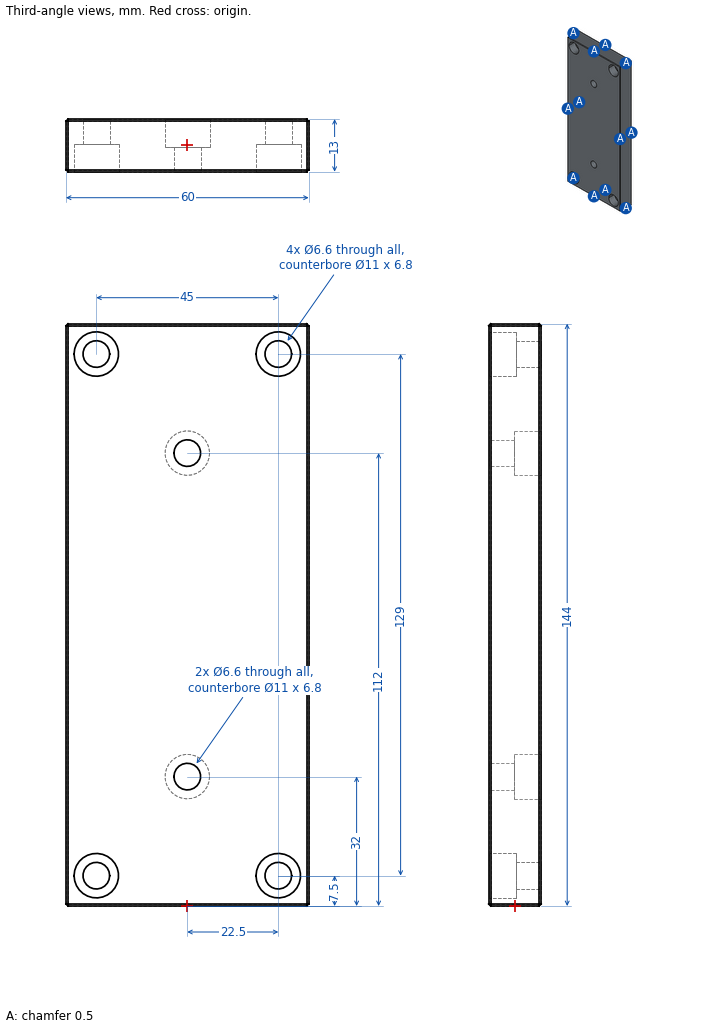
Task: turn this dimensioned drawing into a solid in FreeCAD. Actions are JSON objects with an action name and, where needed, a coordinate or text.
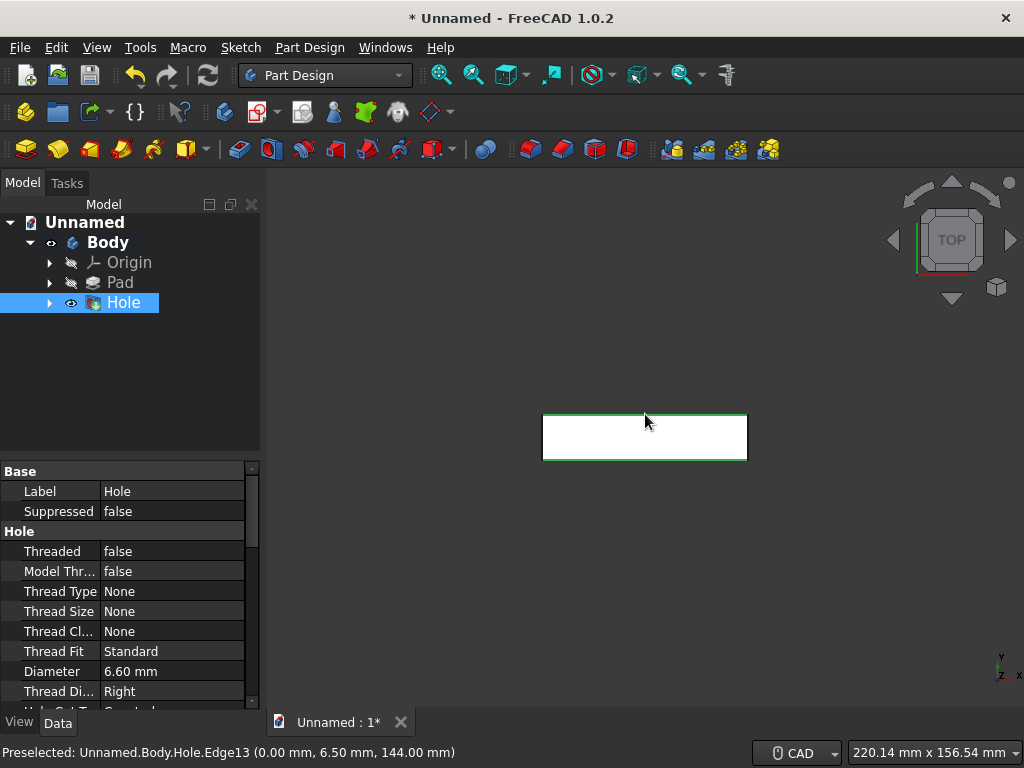
{"action": "key", "text": "1"}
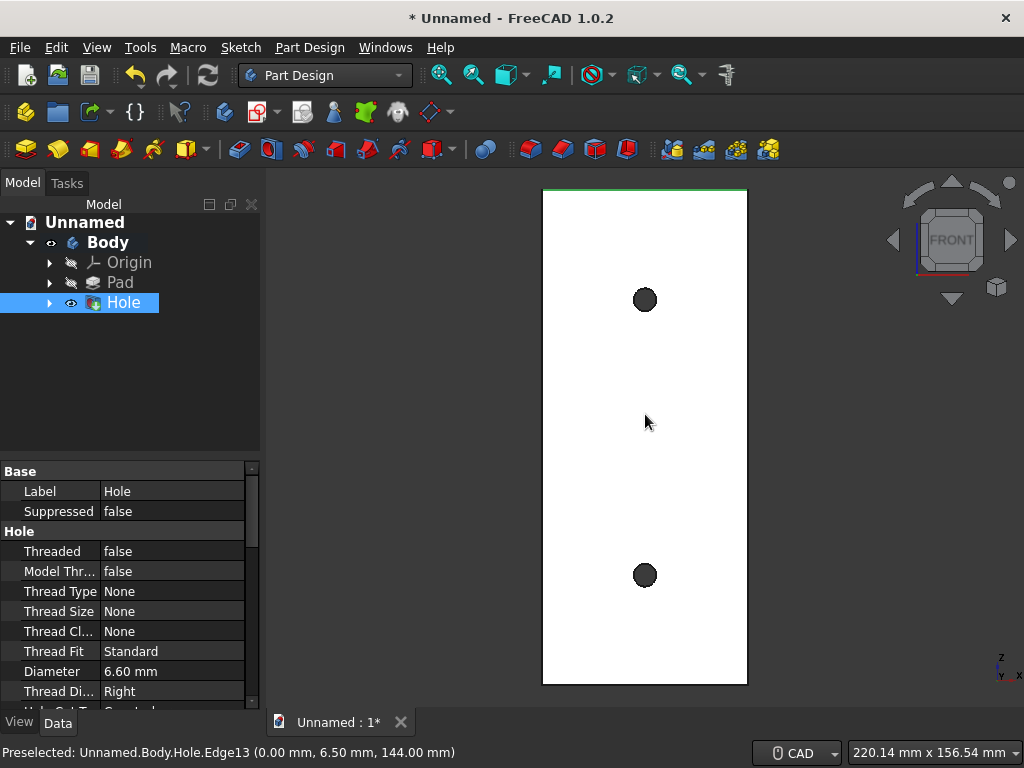
{"action": "key", "text": "3"}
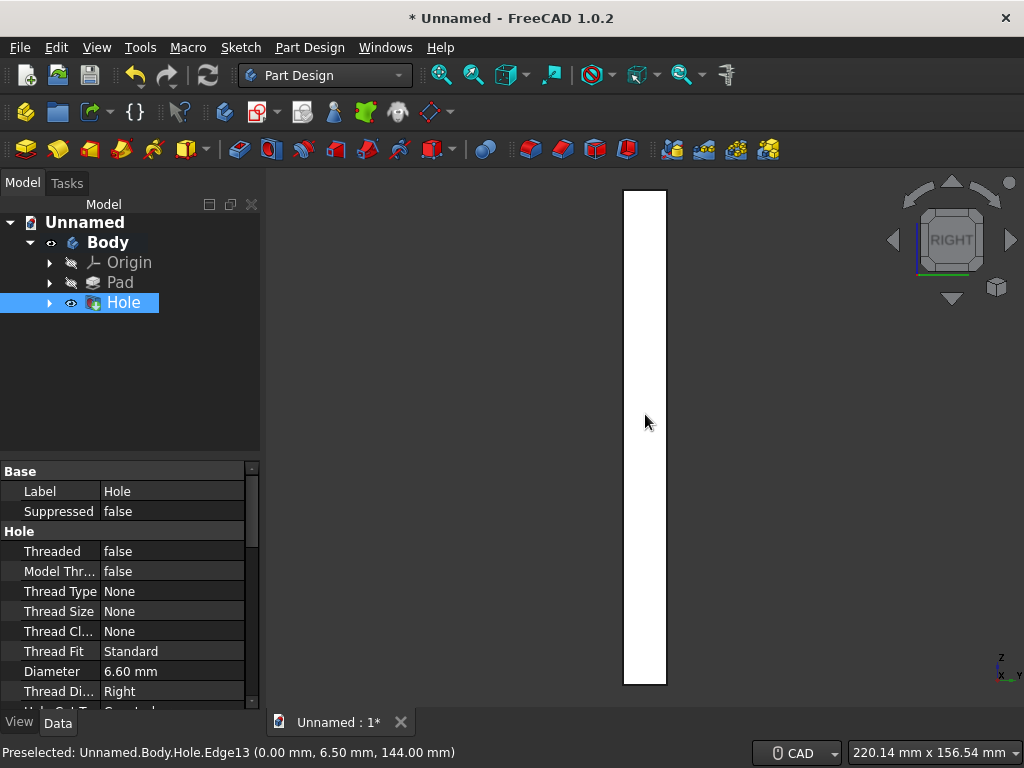
{"action": "key", "text": "5"}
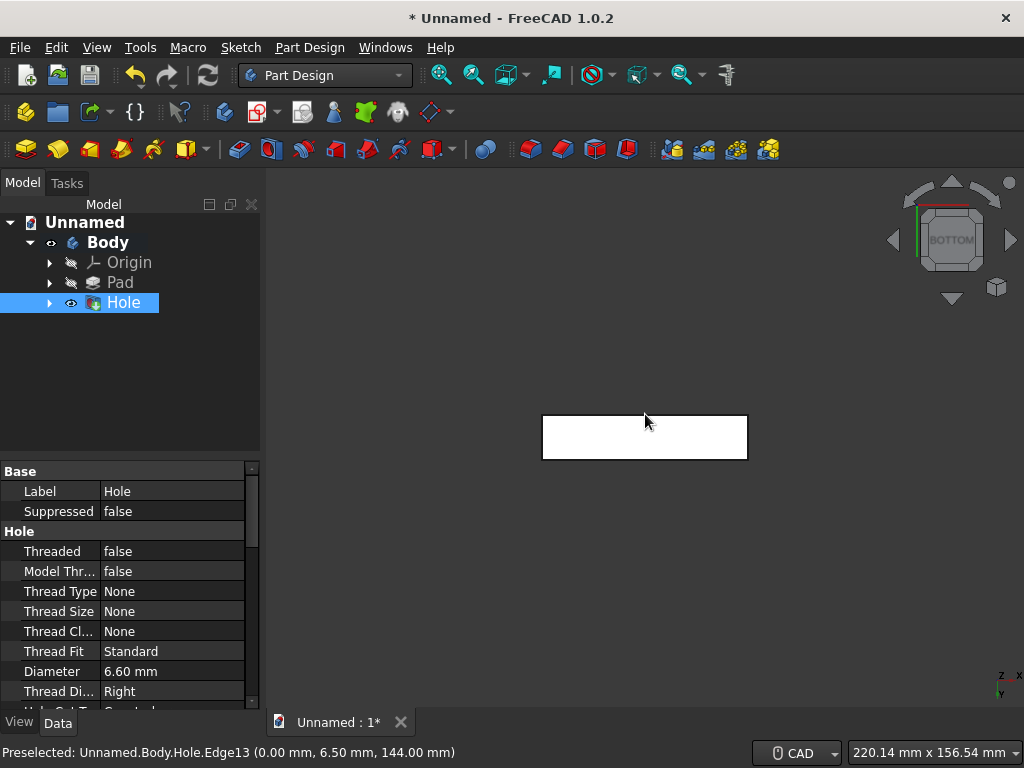
{"action": "key", "text": "v f"}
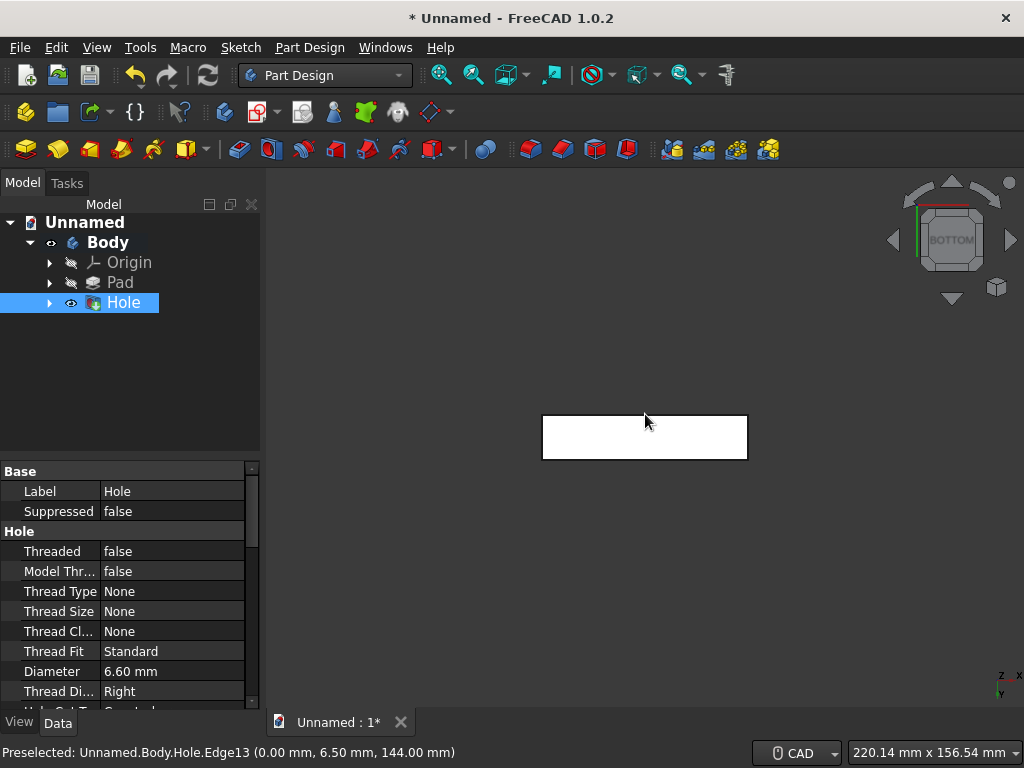
{"action": "left_click", "coordinate": [645, 414], "text": "ctrl"}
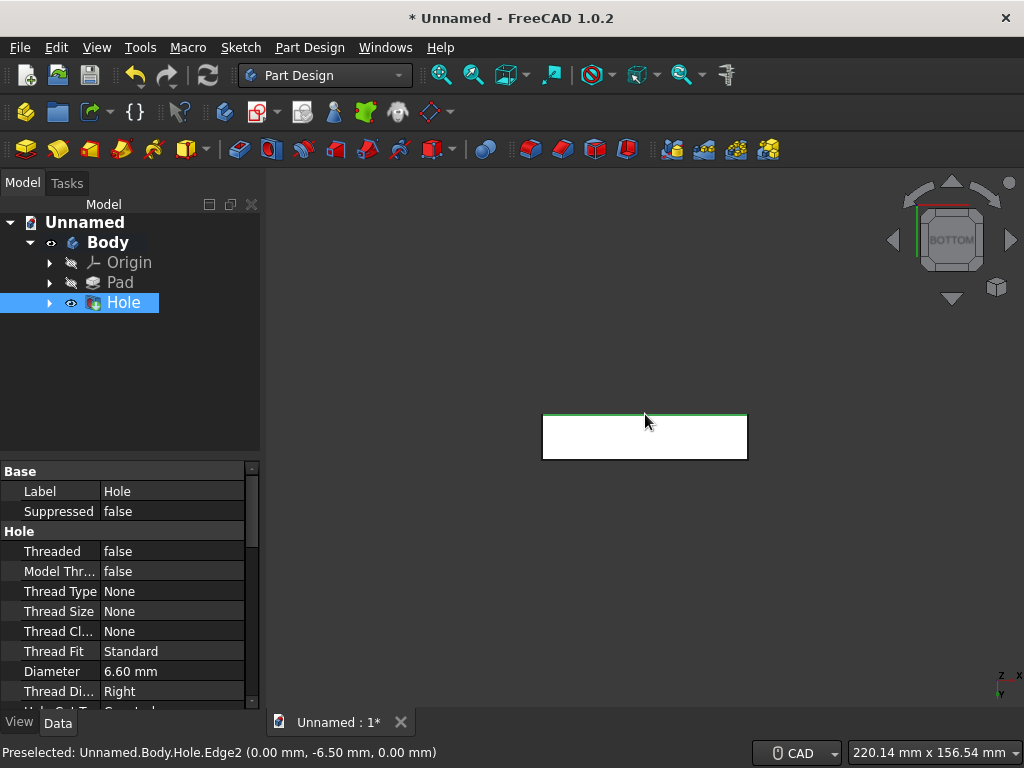
{"action": "left_click", "coordinate": [645, 459], "text": "ctrl"}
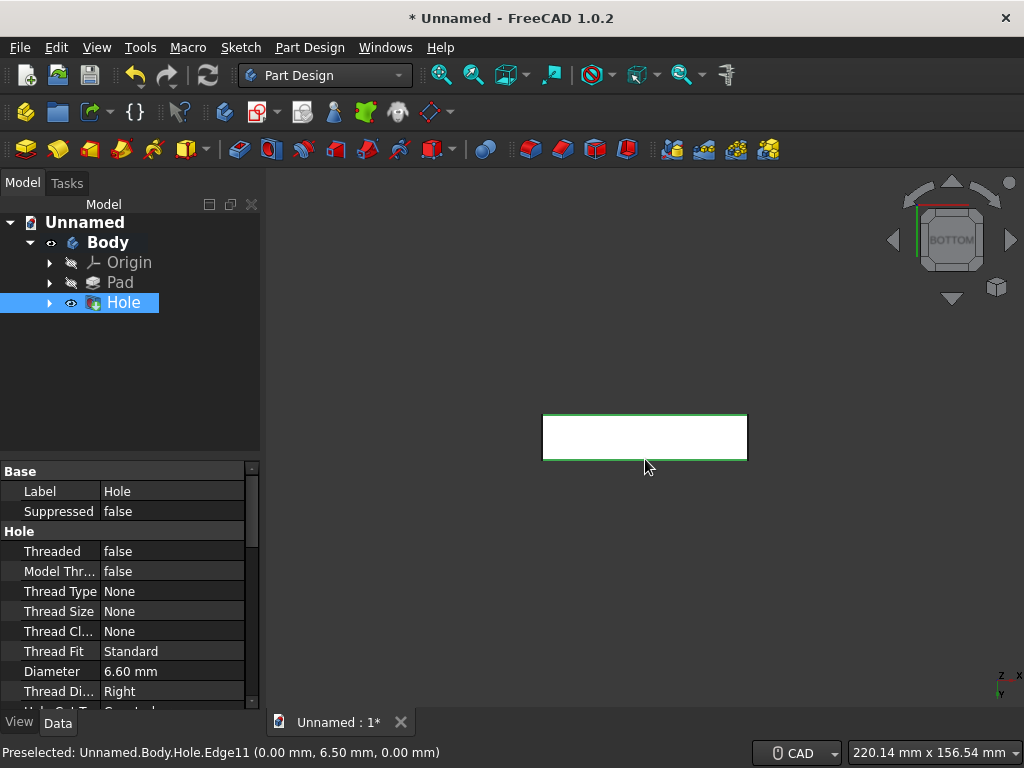
{"action": "key", "text": "4"}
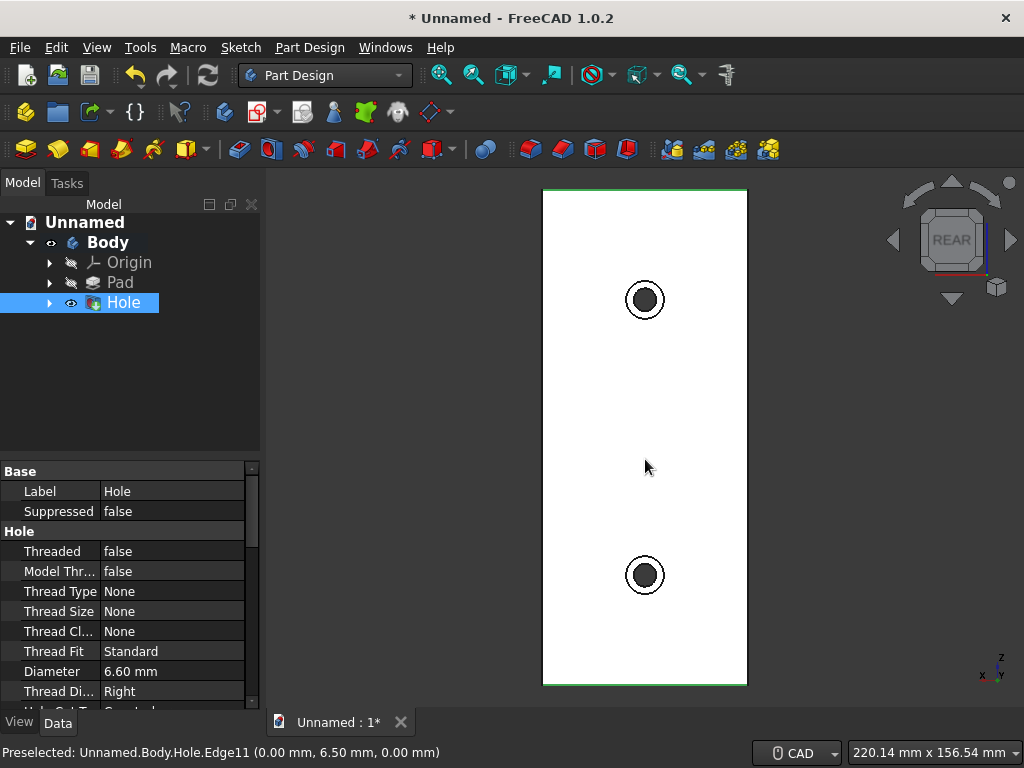
{"action": "key", "text": "6"}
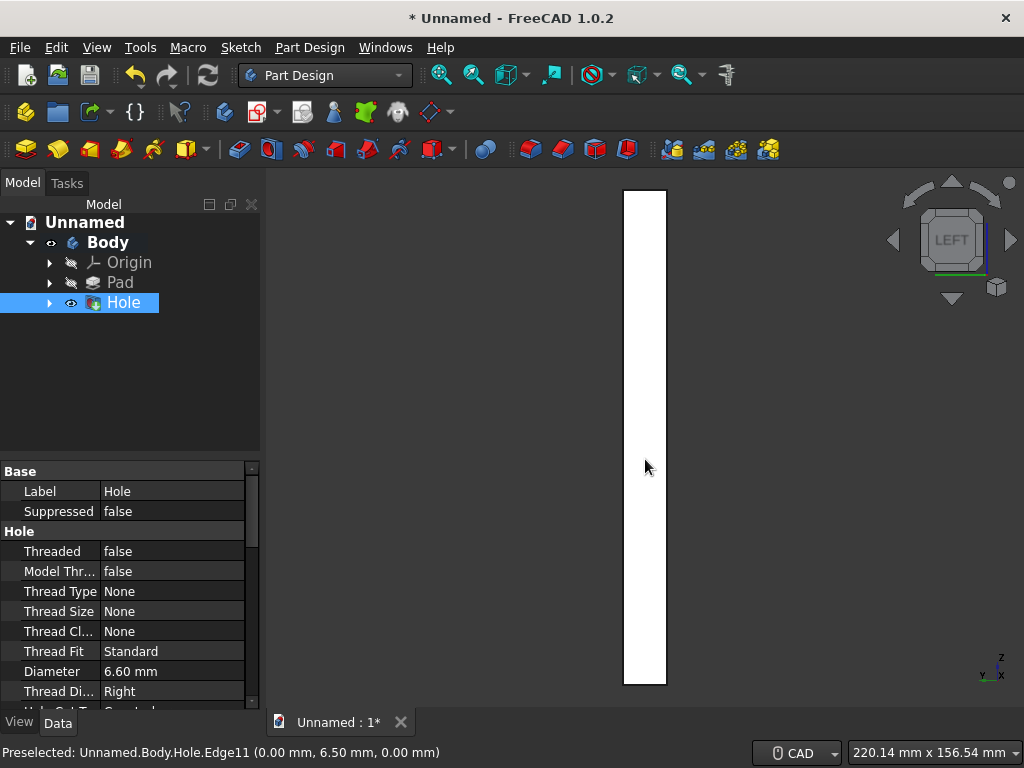
{"action": "left_click", "coordinate": [645, 224], "text": "ctrl"}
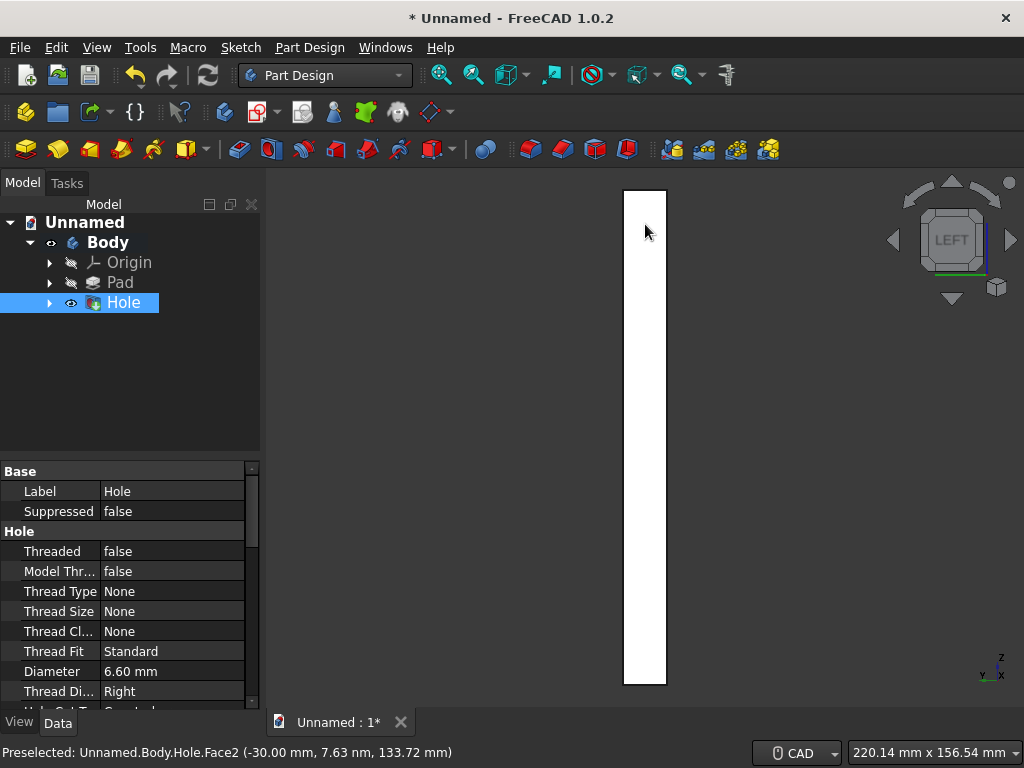
{"action": "left_click", "coordinate": [564, 150]}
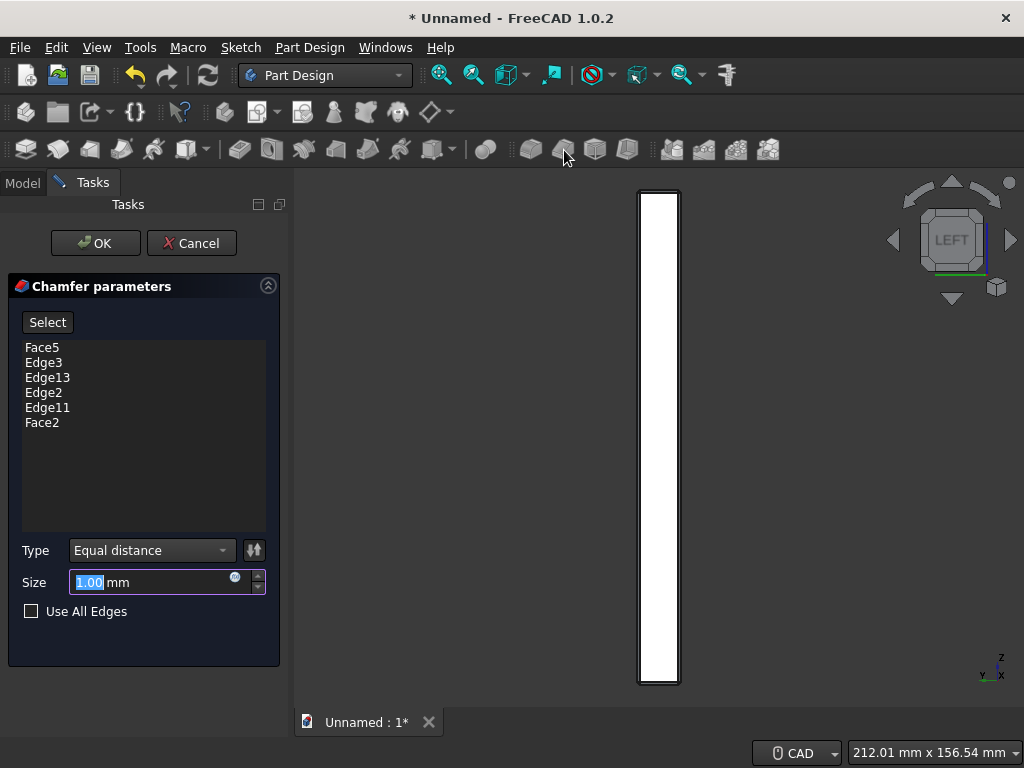
{"action": "type", "text": "0.5"}
{"action": "key", "text": "Tab"}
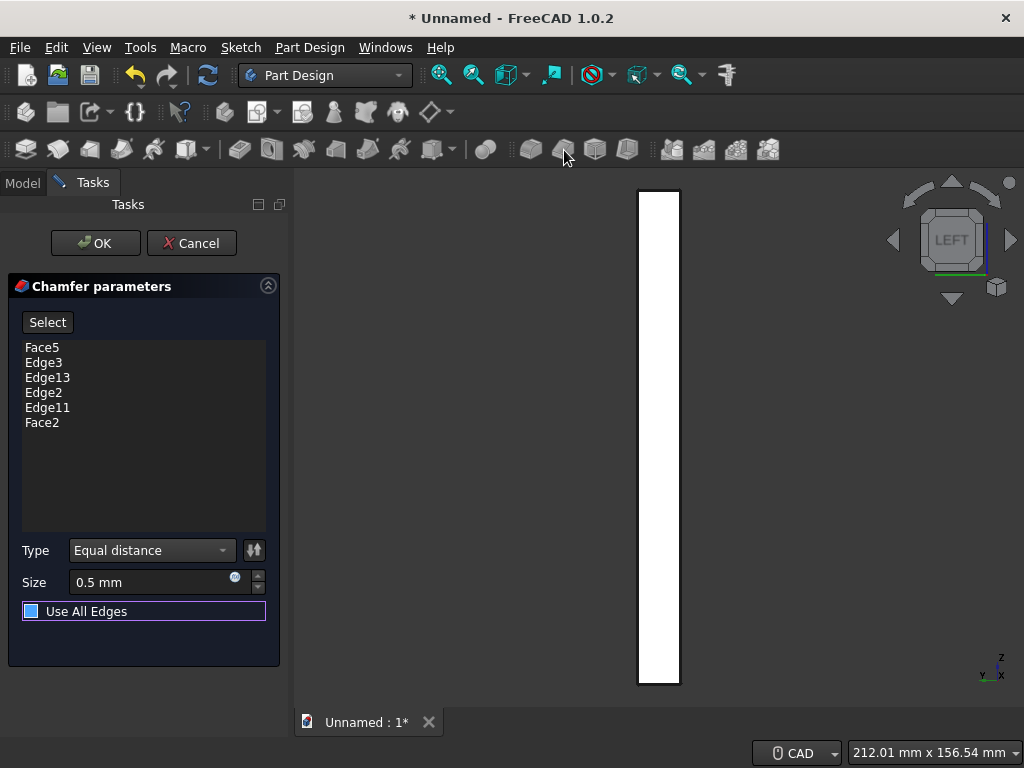
{"action": "left_click", "coordinate": [96, 243]}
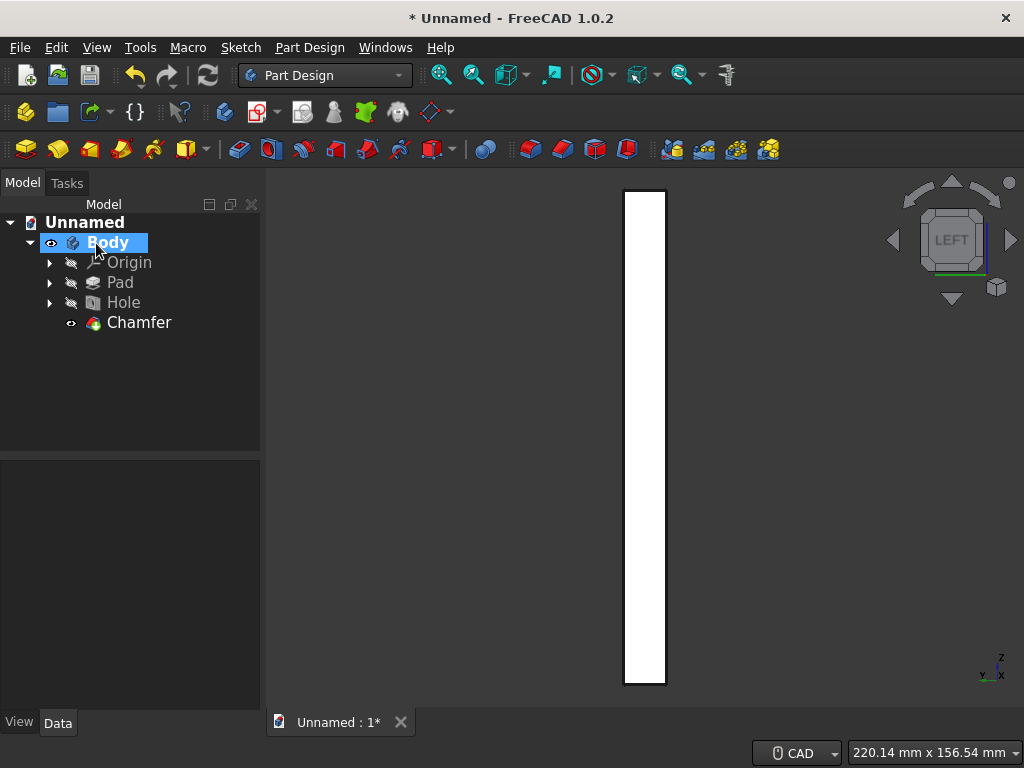
{"action": "key", "text": "0"}